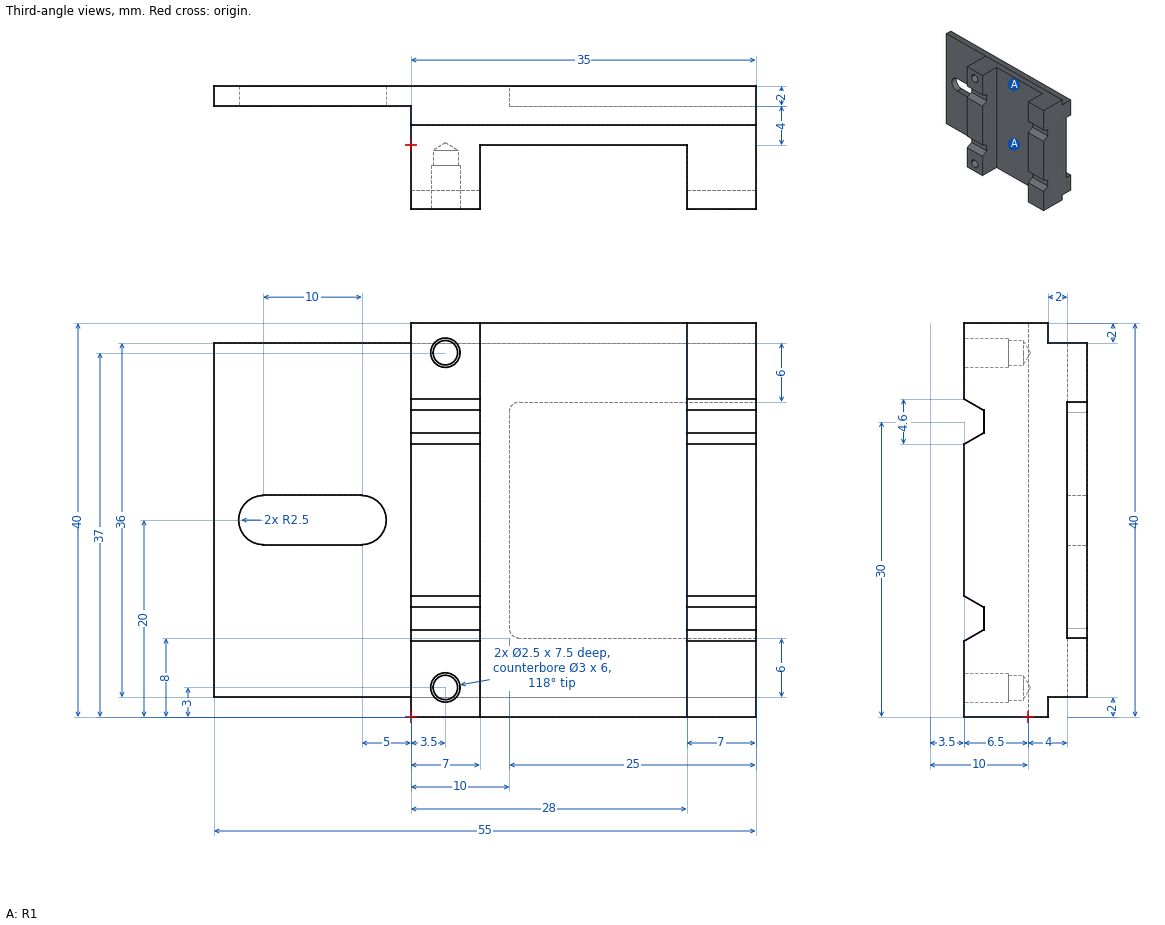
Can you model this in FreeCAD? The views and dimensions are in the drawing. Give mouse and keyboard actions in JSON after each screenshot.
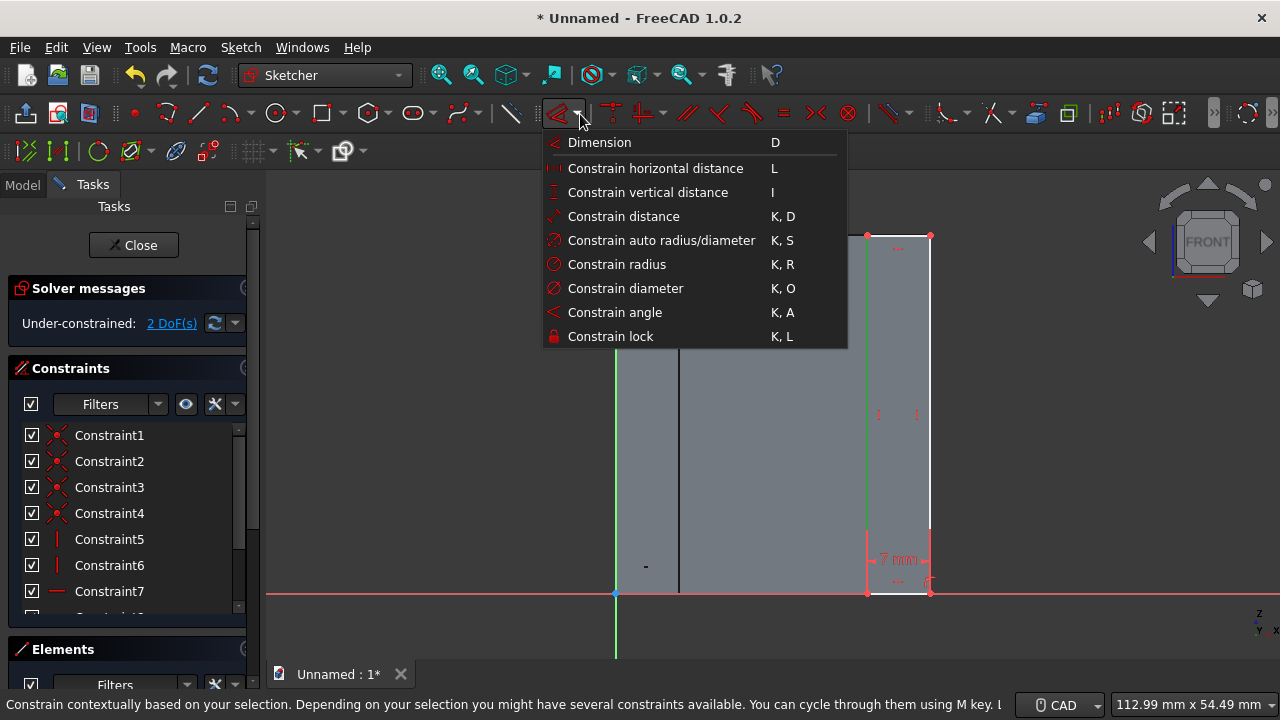
{"action": "left_click", "coordinate": [695, 192]}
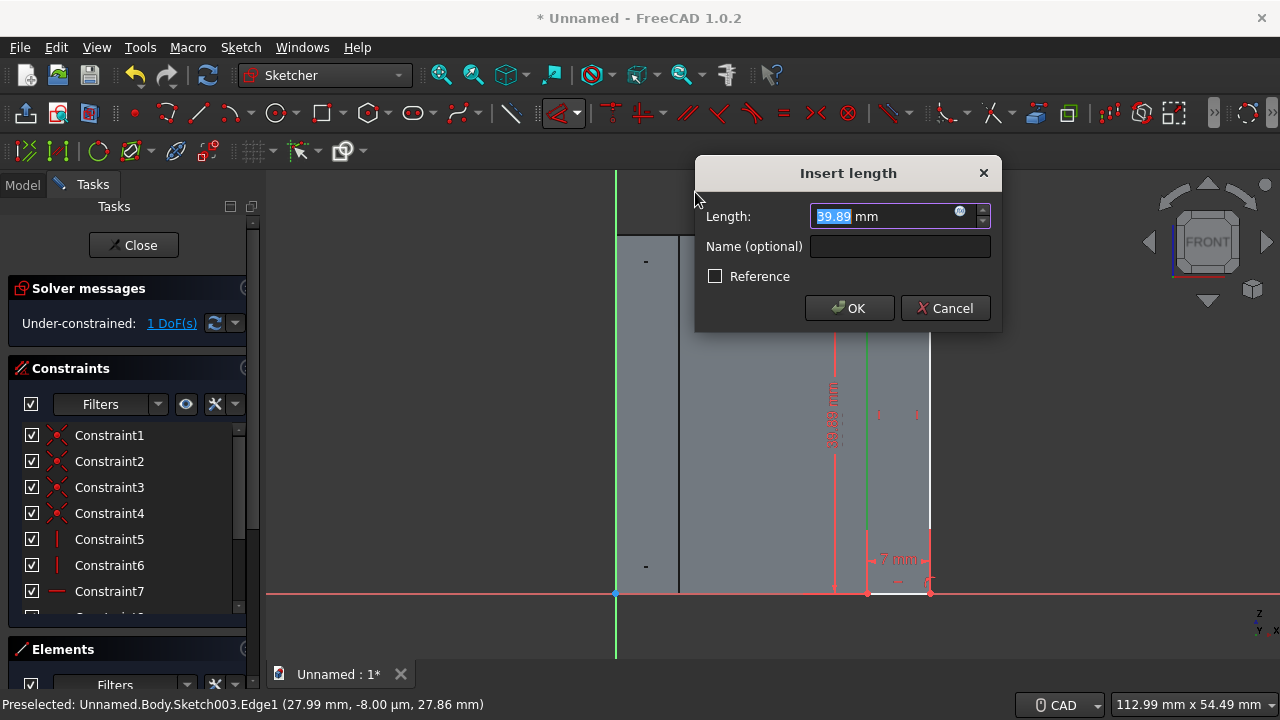
{"action": "type", "text": "40"}
{"action": "key", "text": "Return"}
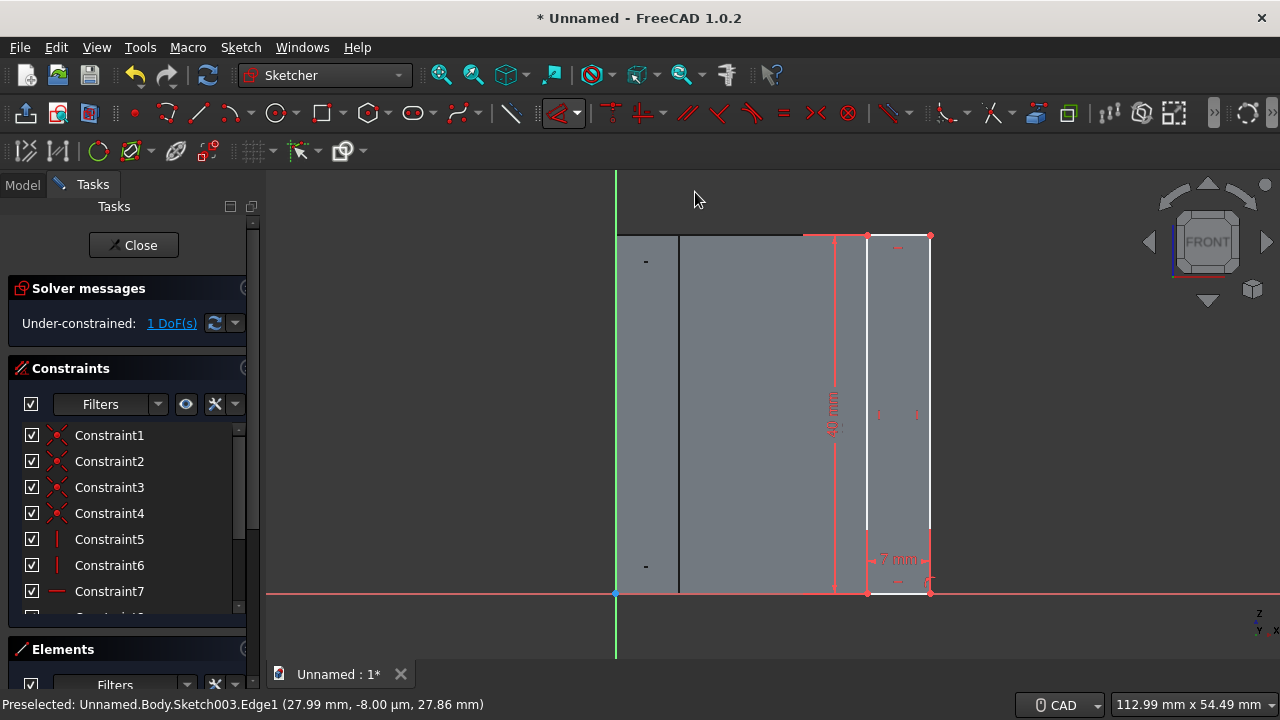
{"action": "left_click", "coordinate": [867, 235]}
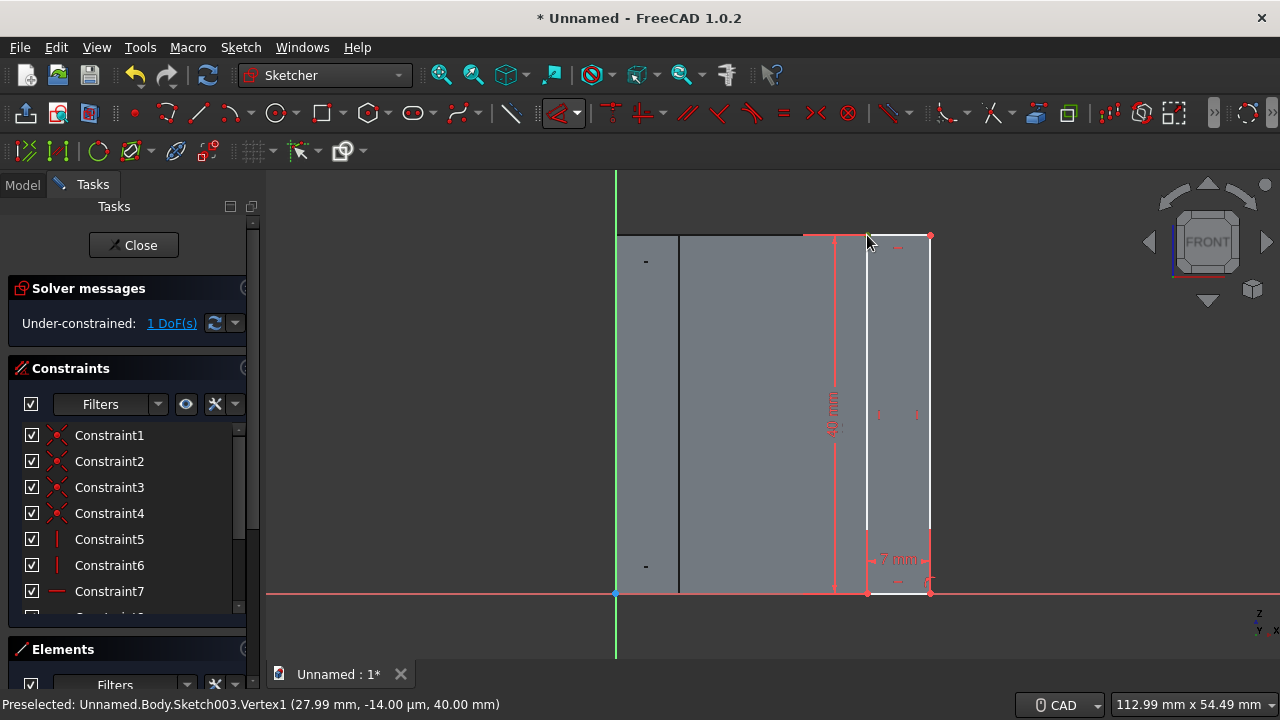
{"action": "left_click", "coordinate": [580, 114]}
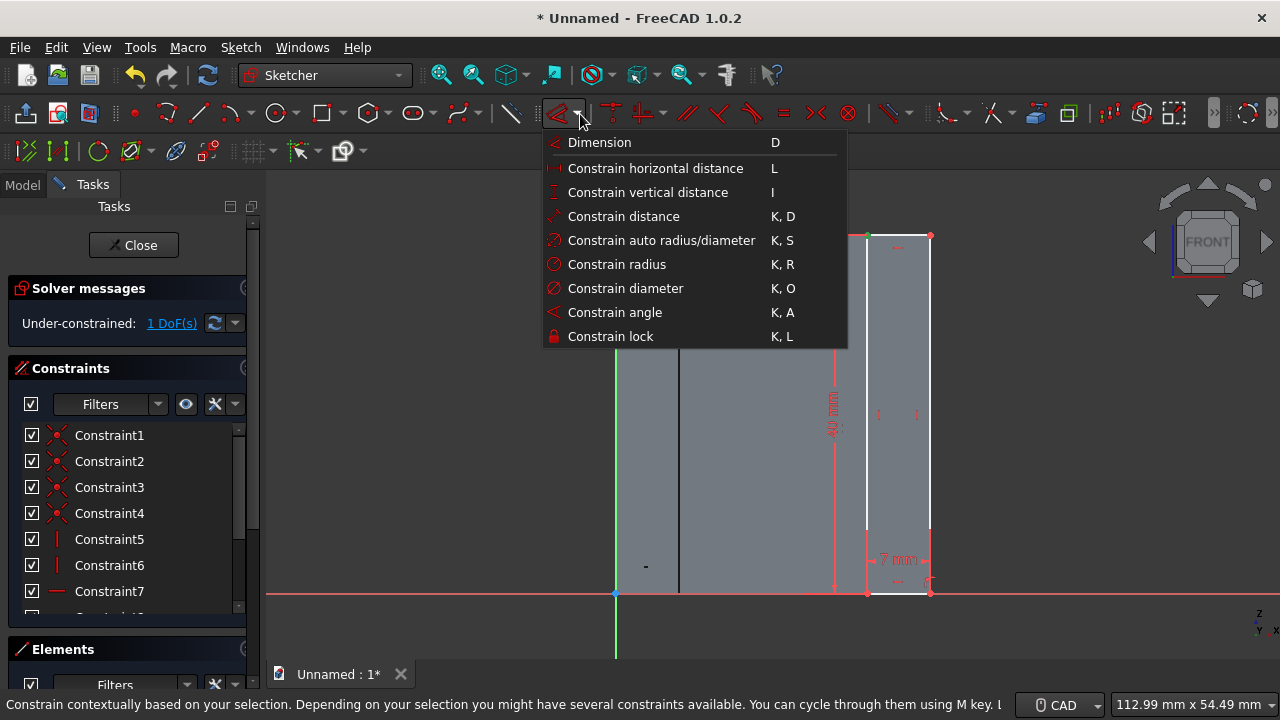
{"action": "left_click", "coordinate": [695, 168]}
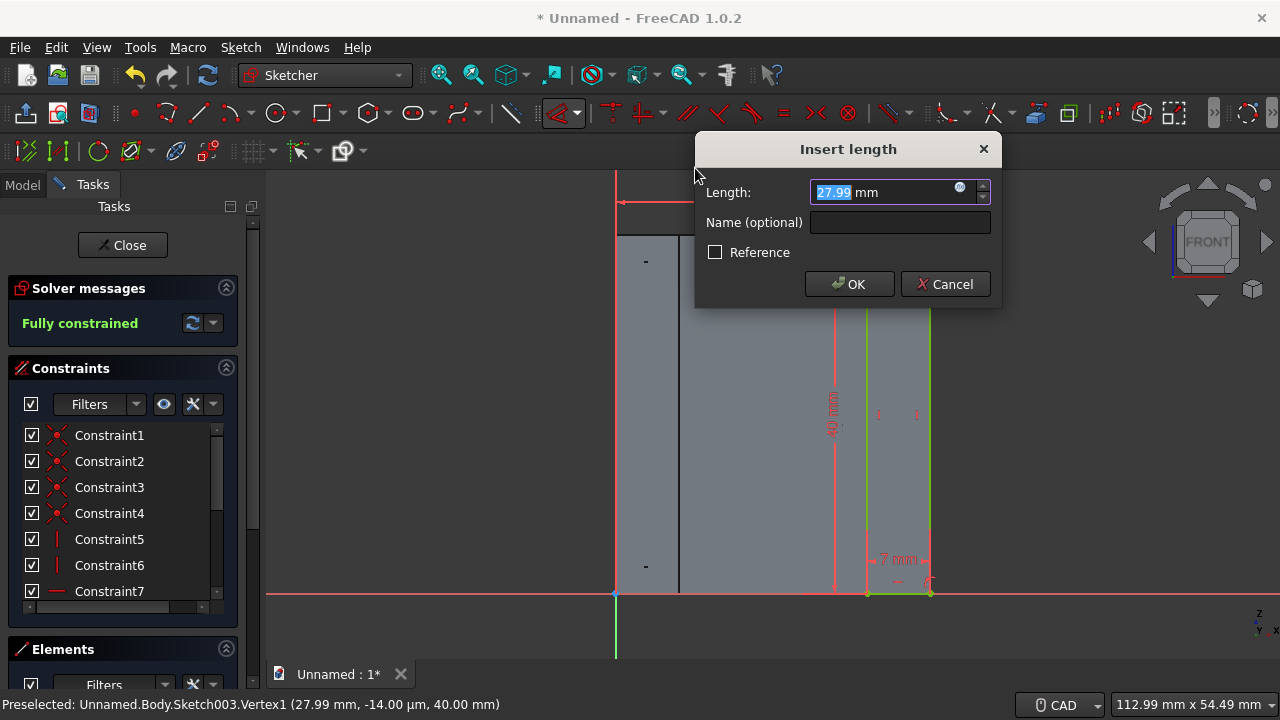
{"action": "type", "text": "28"}
{"action": "key", "text": "Return"}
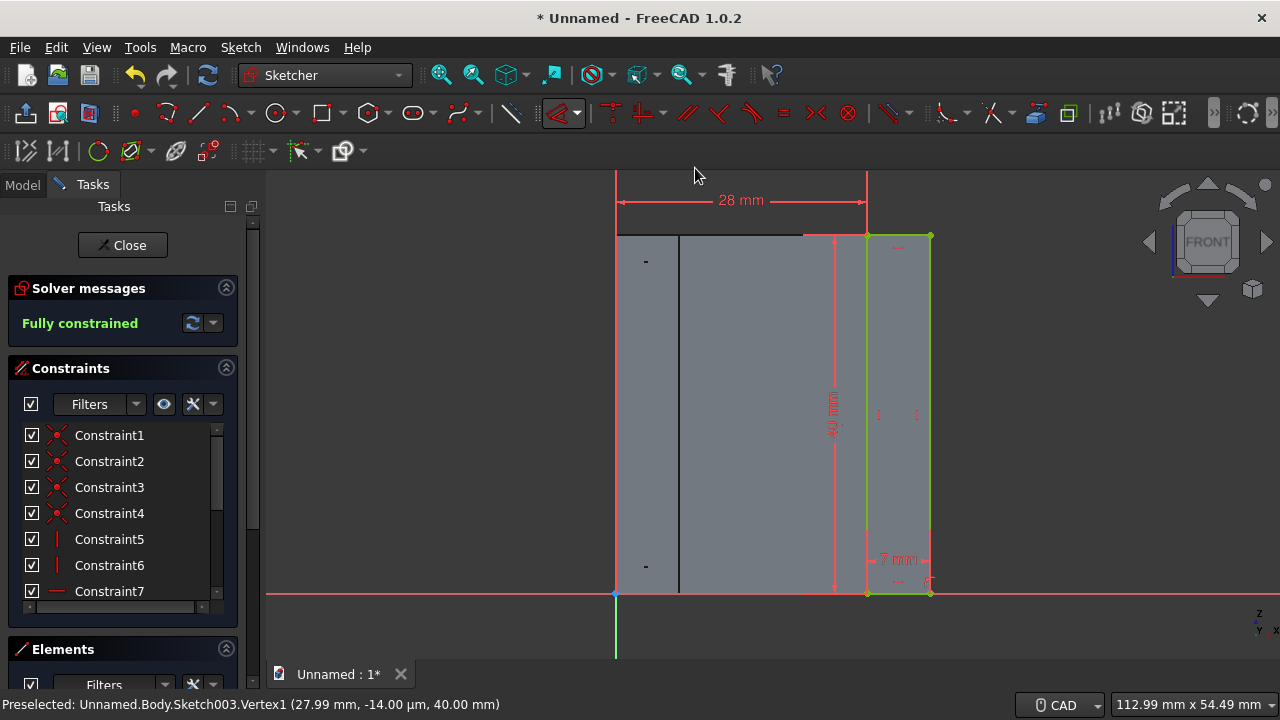
{"action": "left_click", "coordinate": [123, 245]}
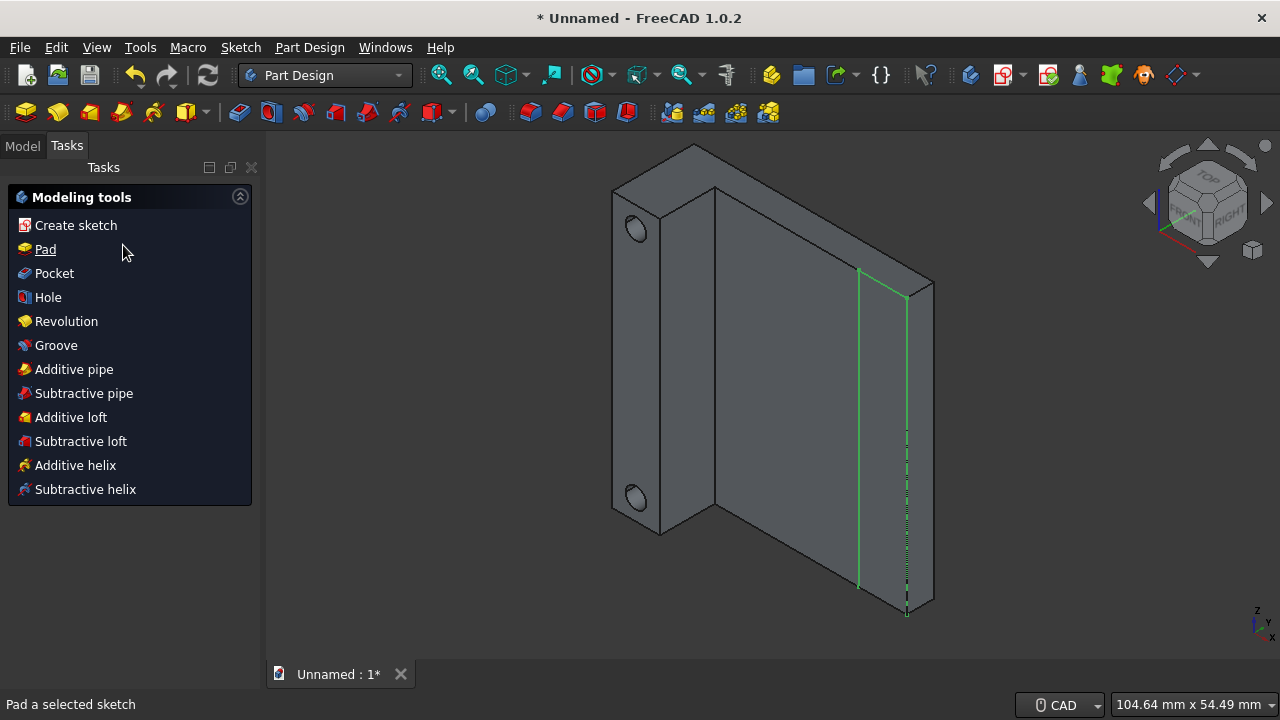
{"action": "left_click", "coordinate": [26, 112]}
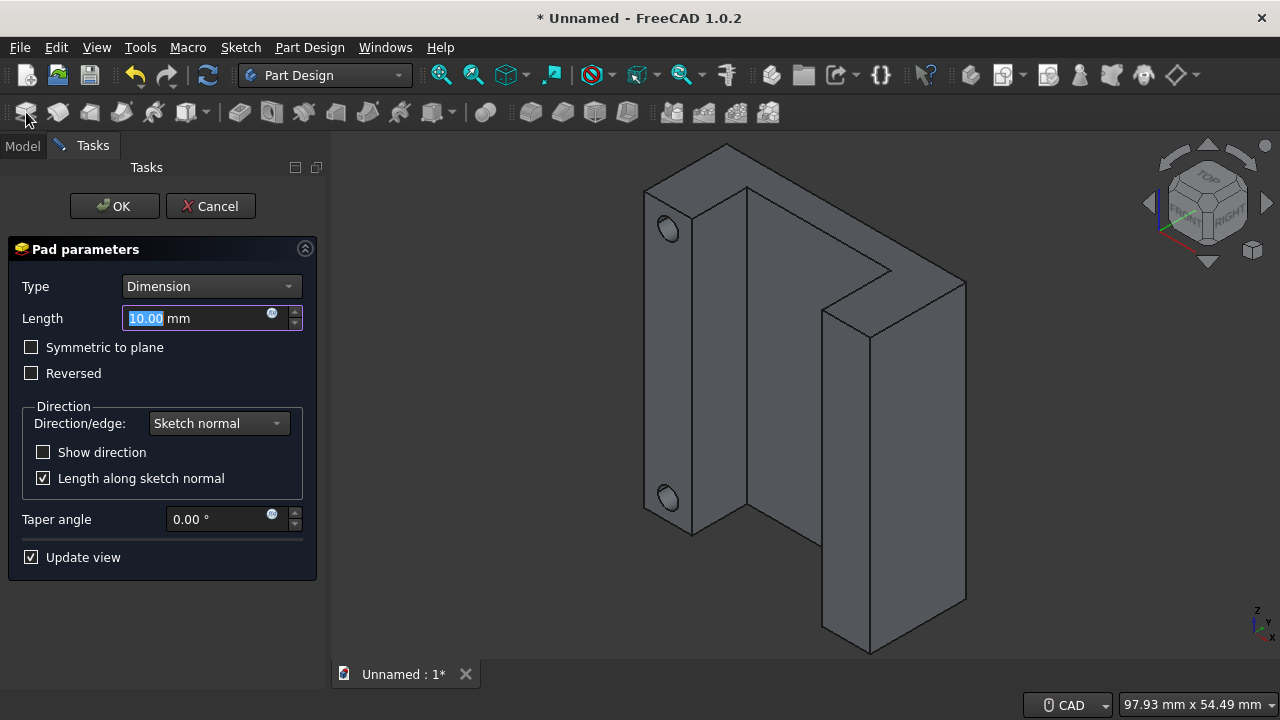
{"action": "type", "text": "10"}
{"action": "key", "text": "Tab"}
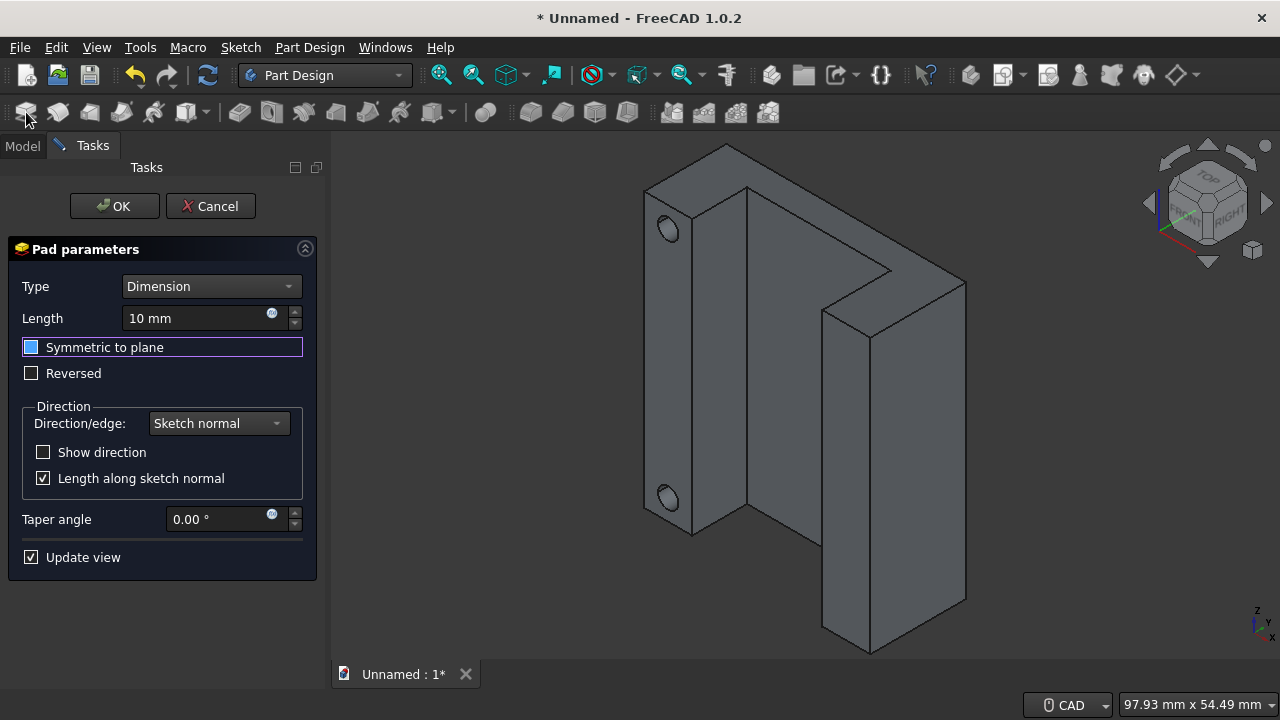
{"action": "left_click", "coordinate": [115, 206]}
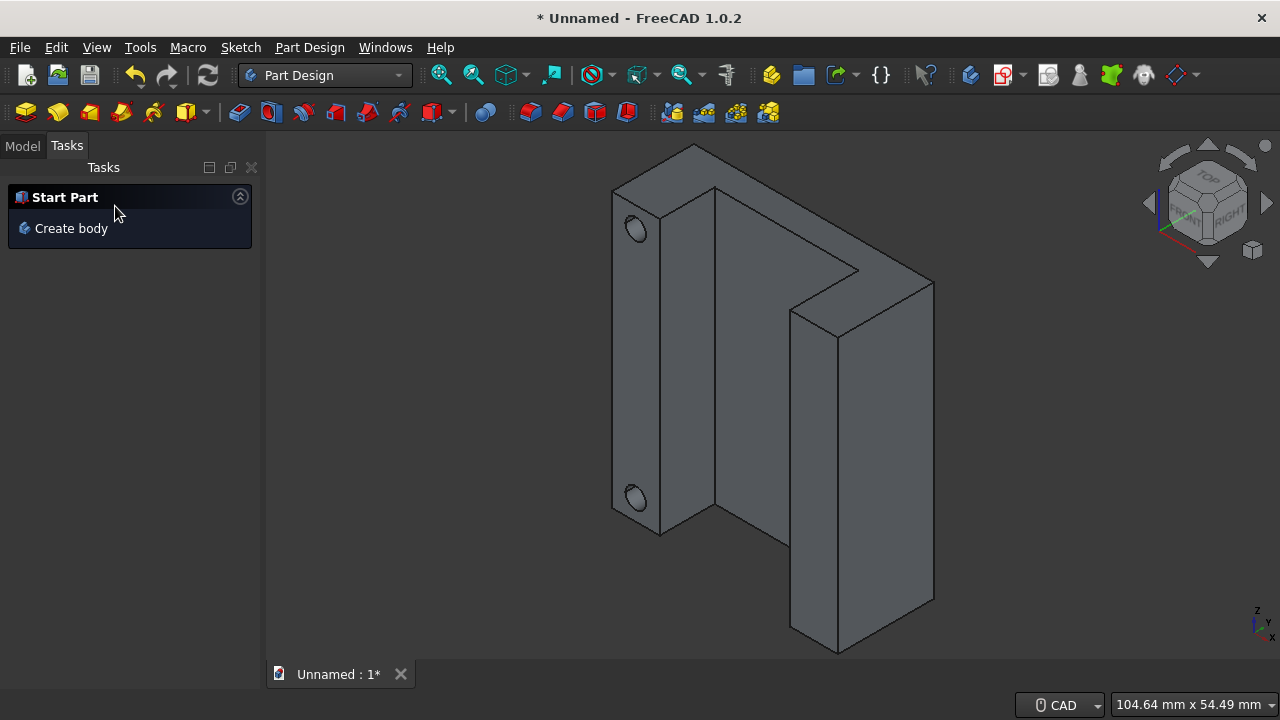
{"action": "left_click", "coordinate": [886, 558]}